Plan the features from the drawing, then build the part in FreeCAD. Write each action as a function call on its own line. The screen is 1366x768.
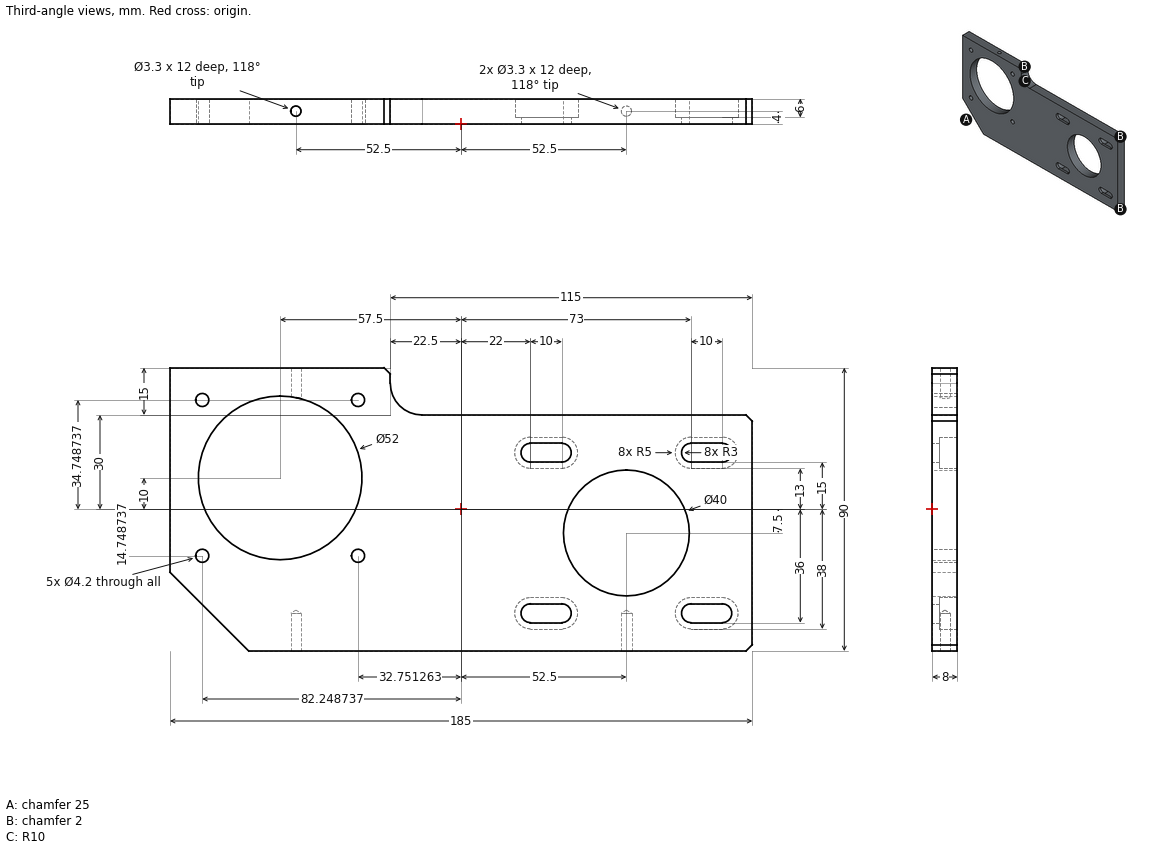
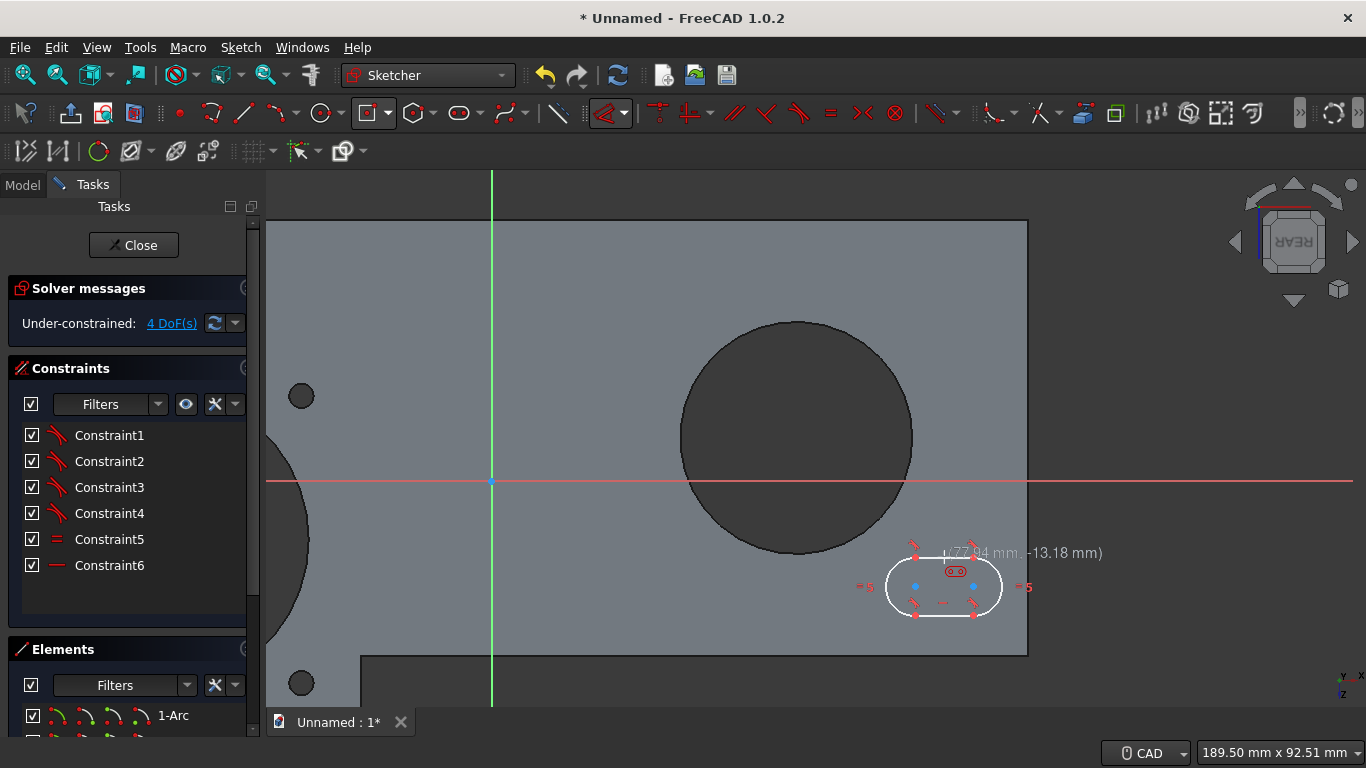
click(915, 290)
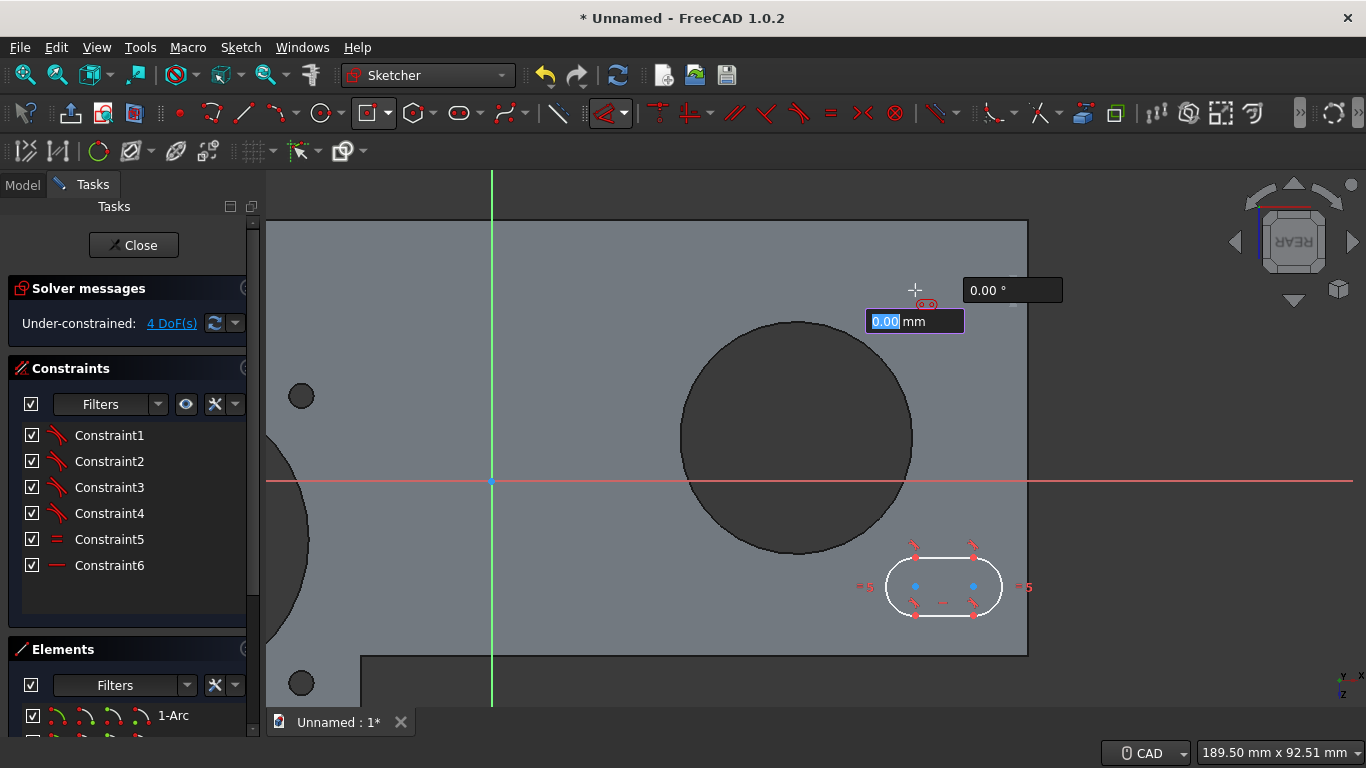
click(973, 290)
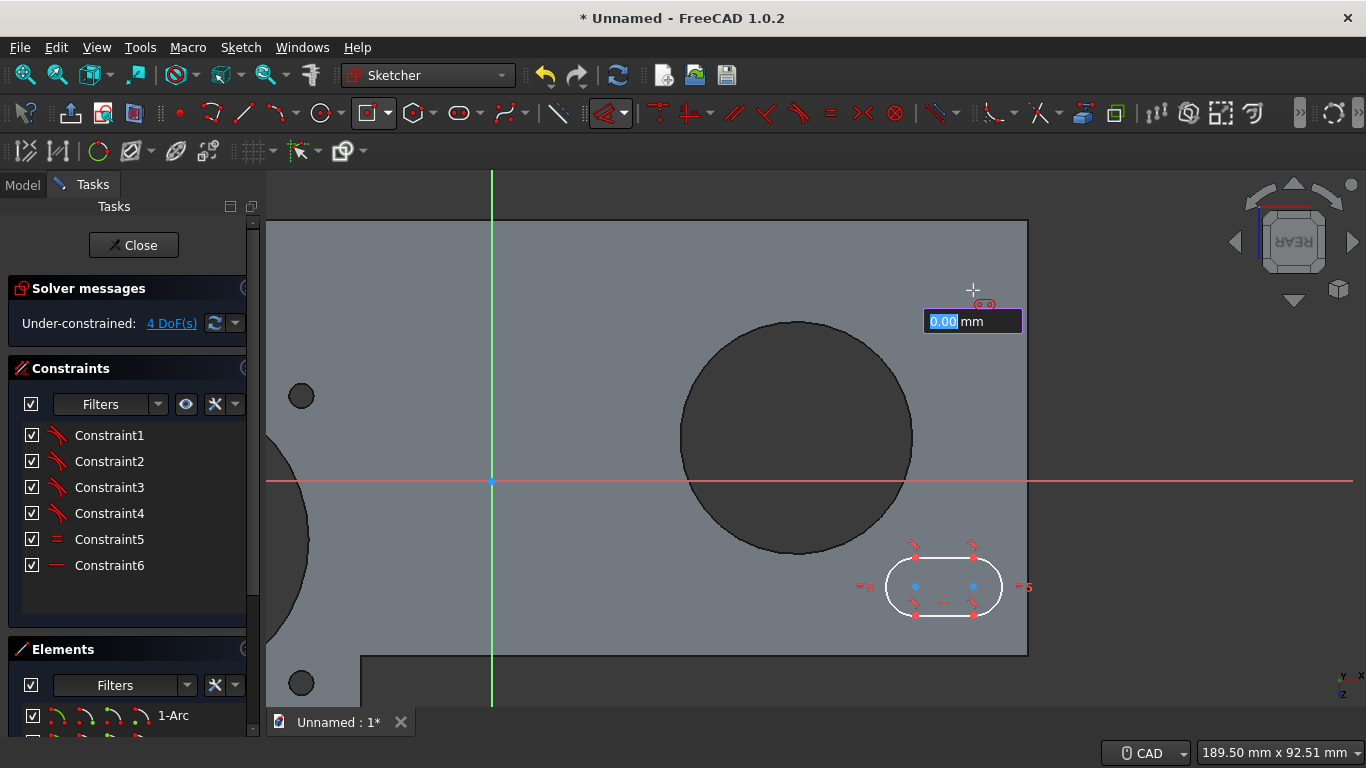
click(944, 319)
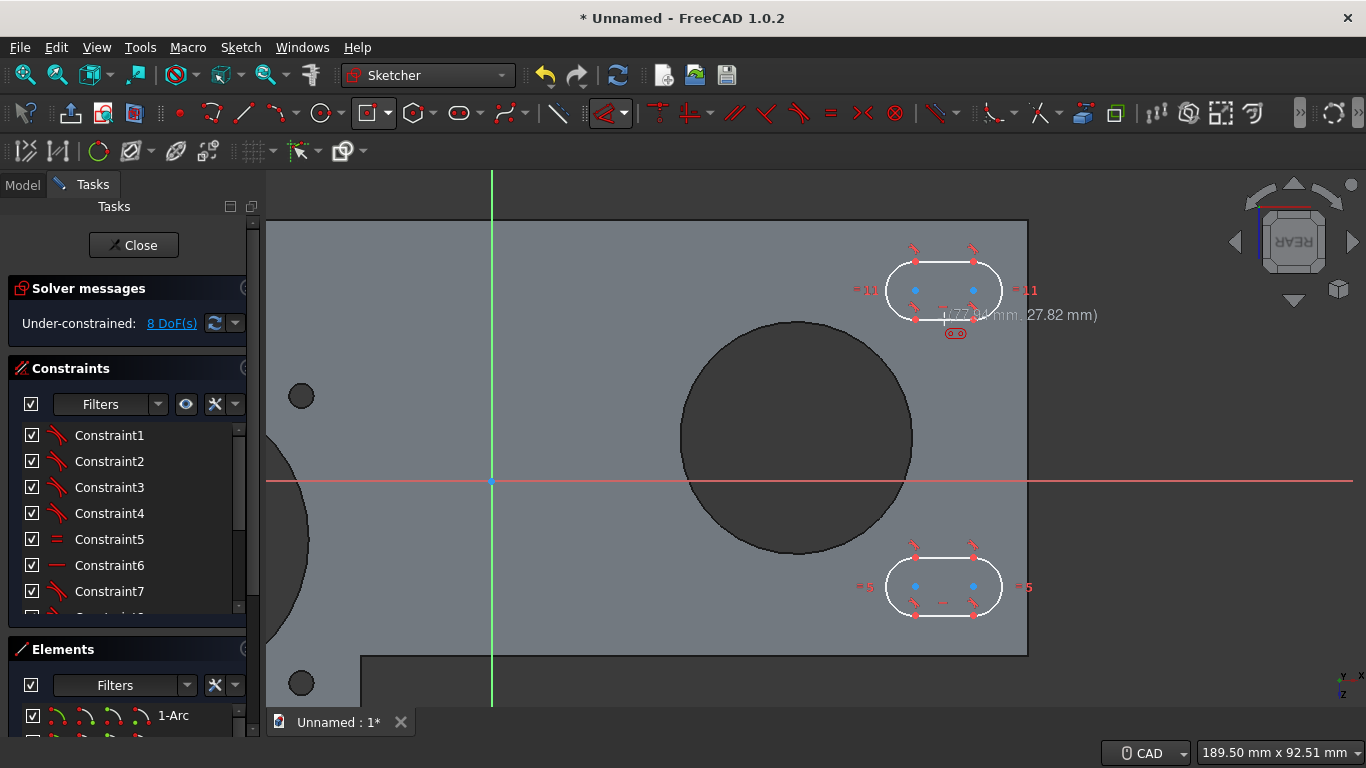
click(619, 586)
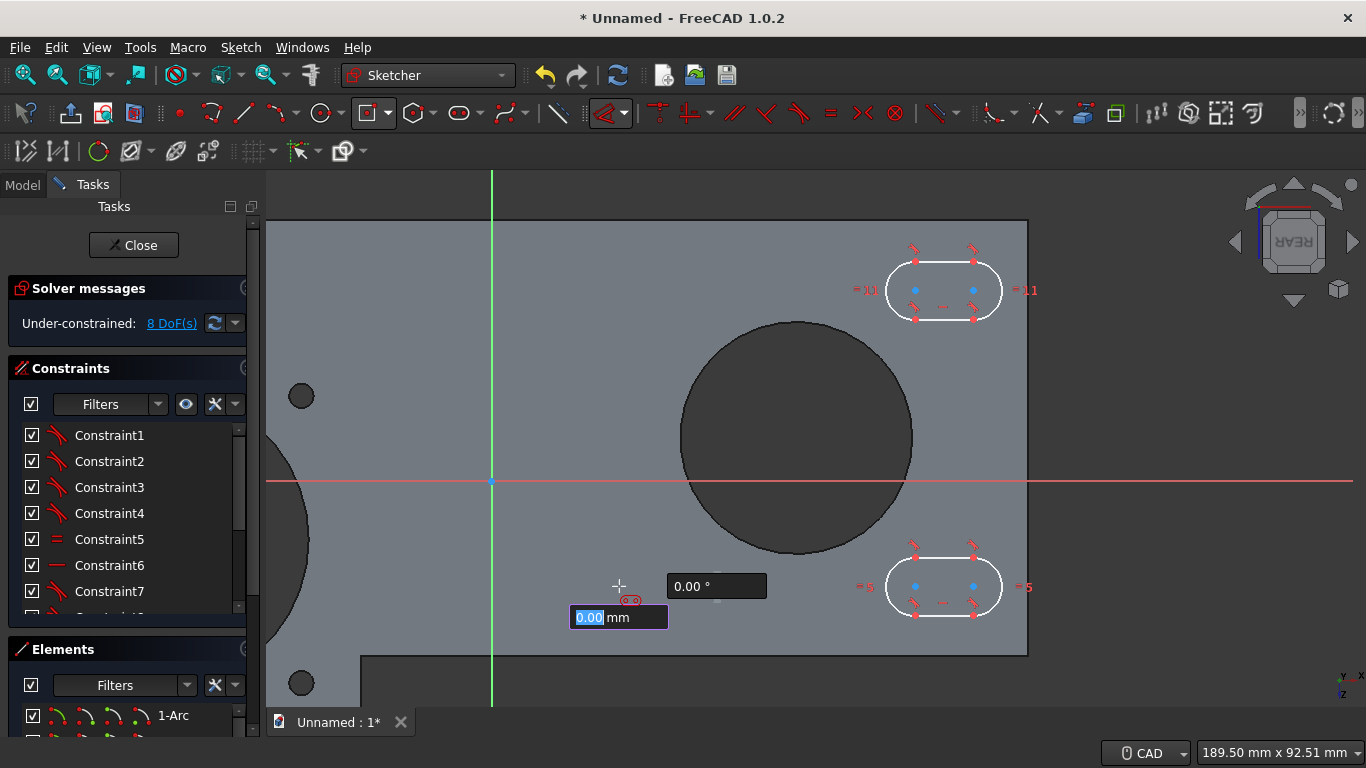
click(677, 586)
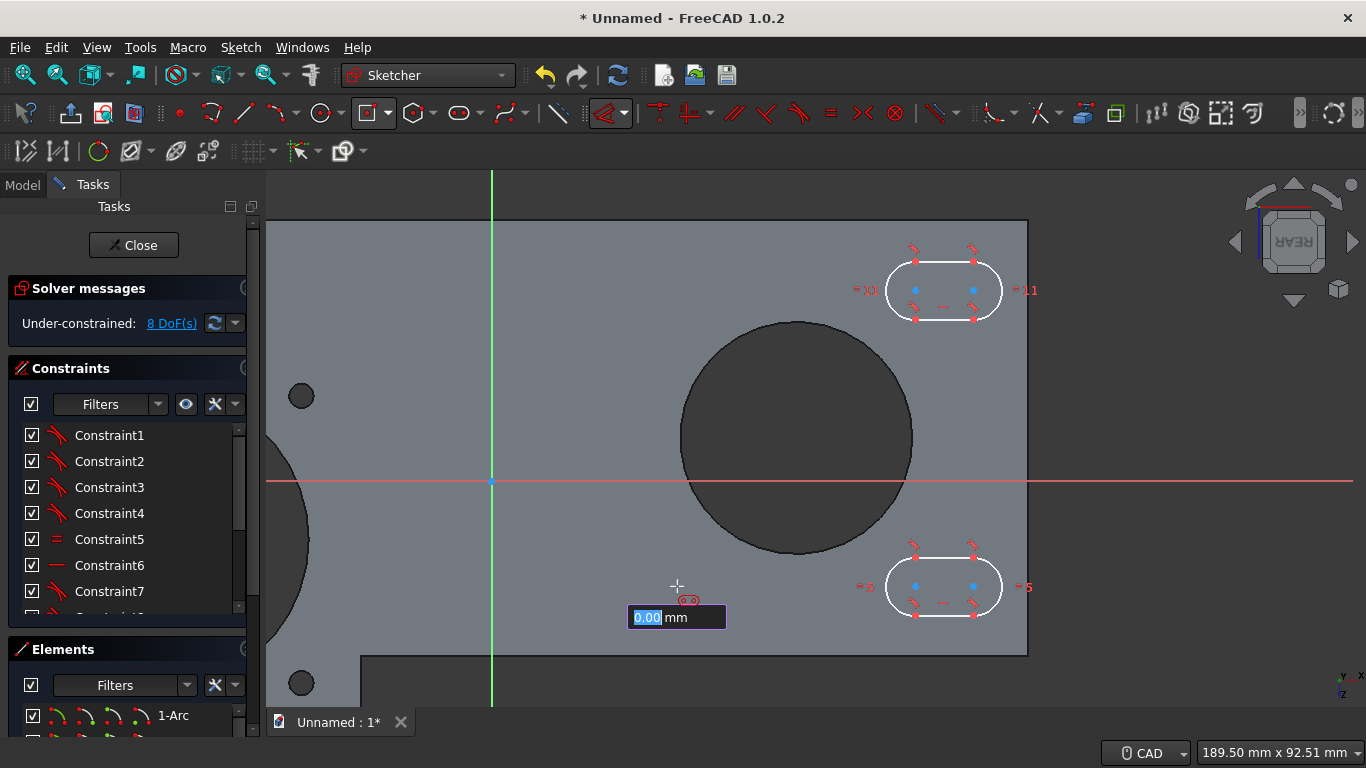
click(648, 557)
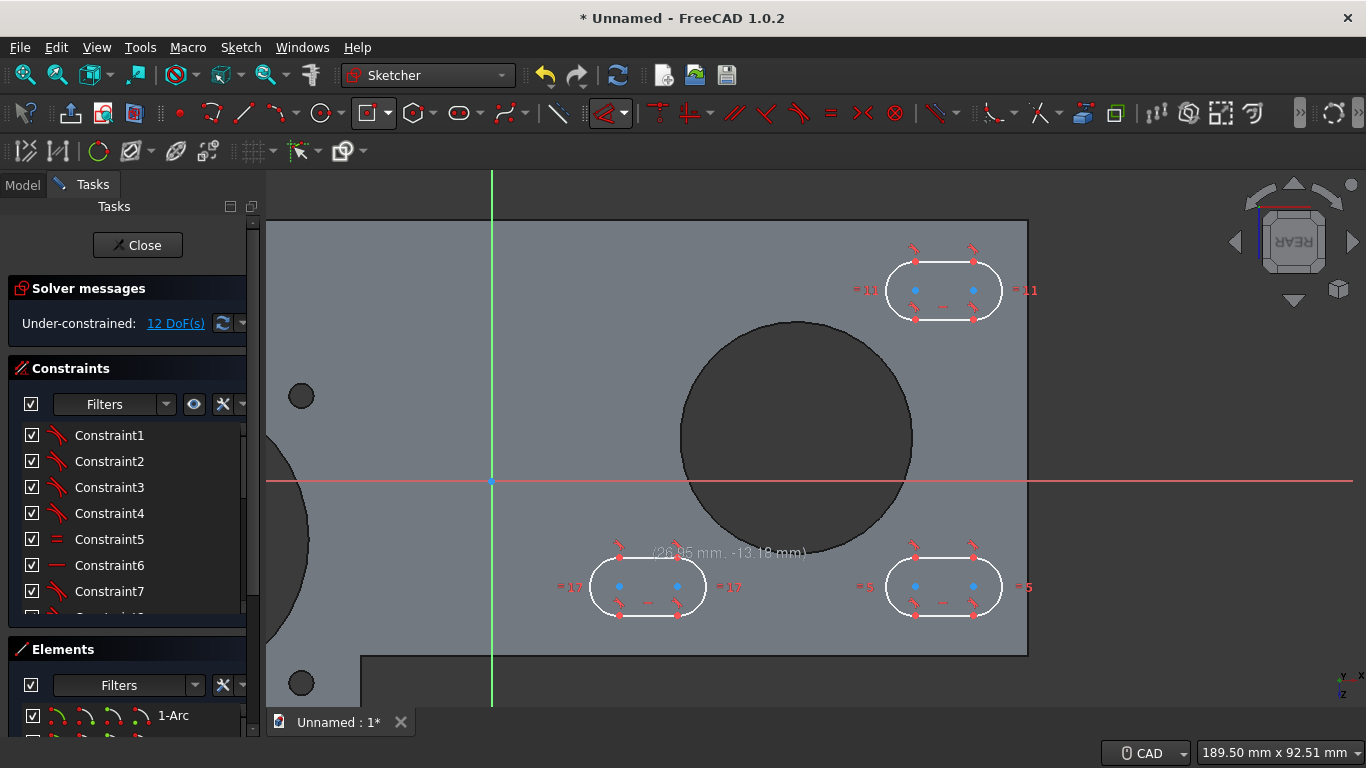
click(619, 290)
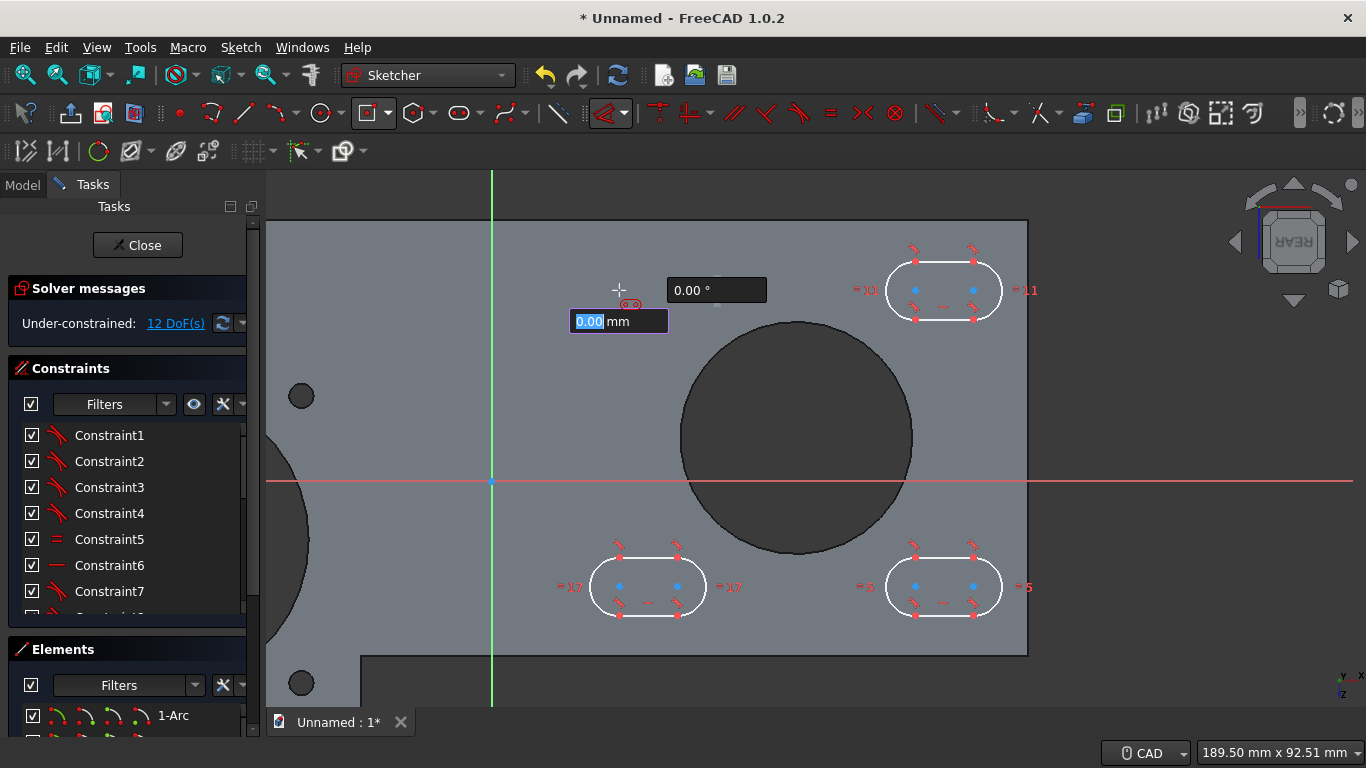
click(677, 290)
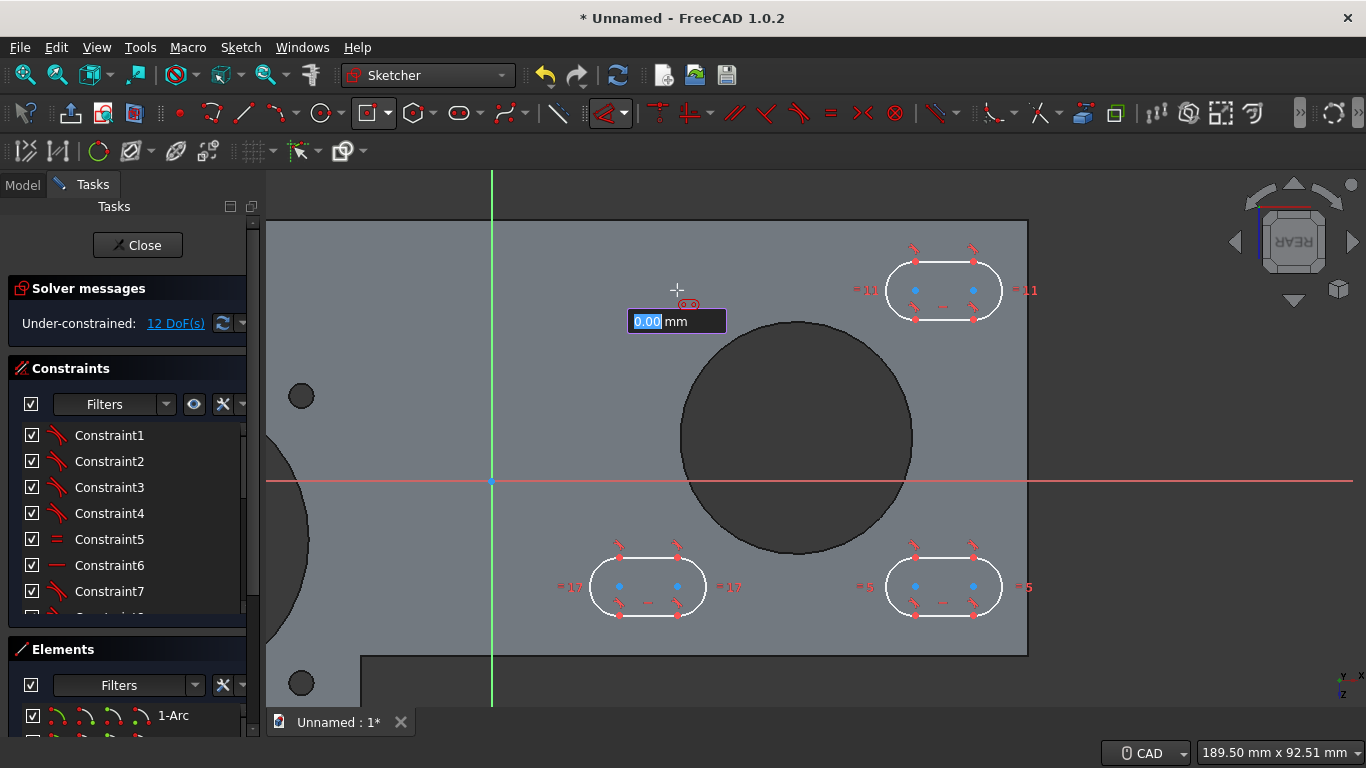
click(648, 319)
key(Escape)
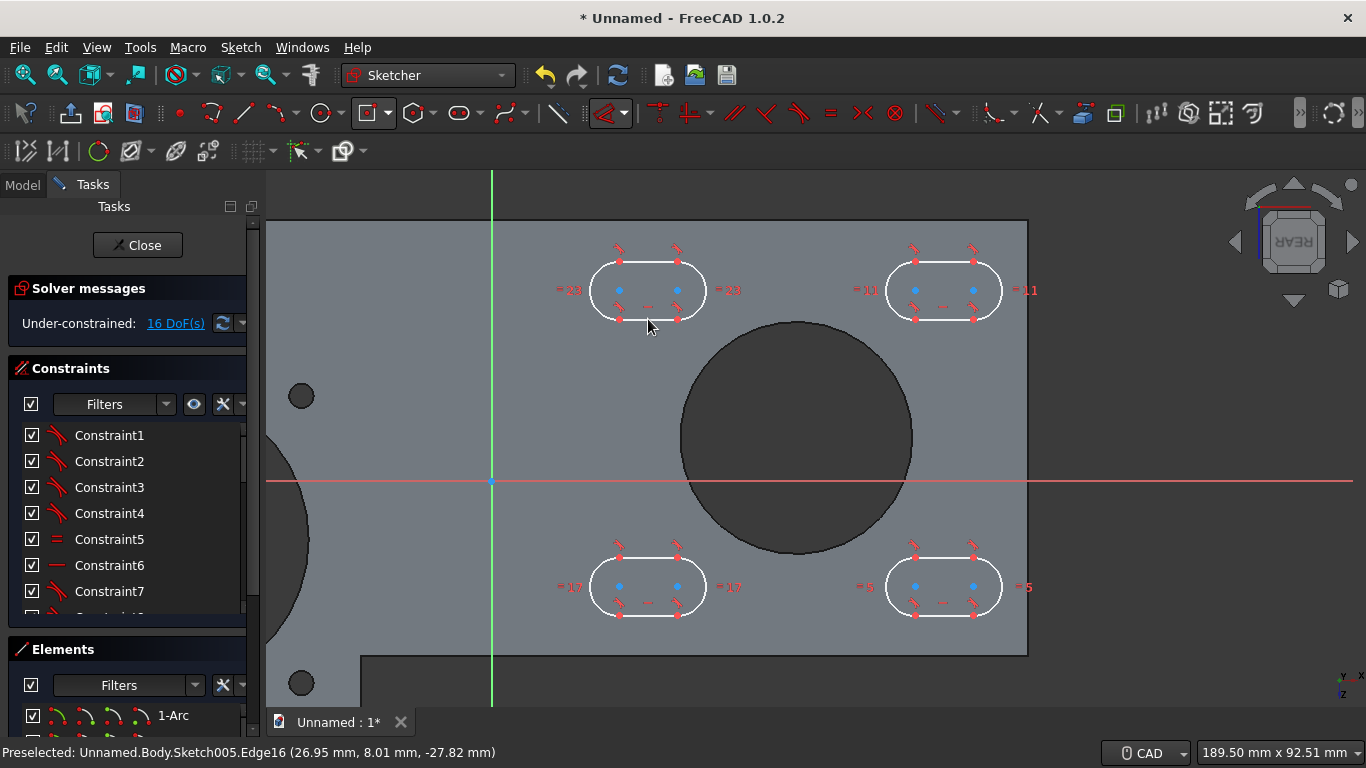
click(892, 570)